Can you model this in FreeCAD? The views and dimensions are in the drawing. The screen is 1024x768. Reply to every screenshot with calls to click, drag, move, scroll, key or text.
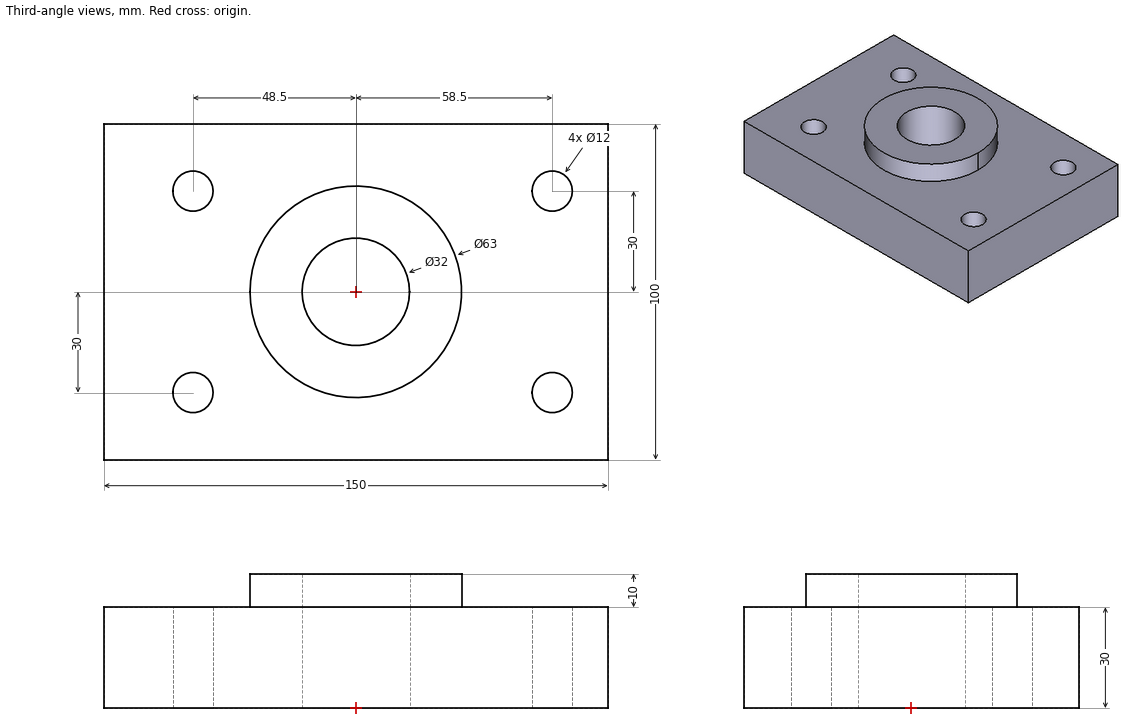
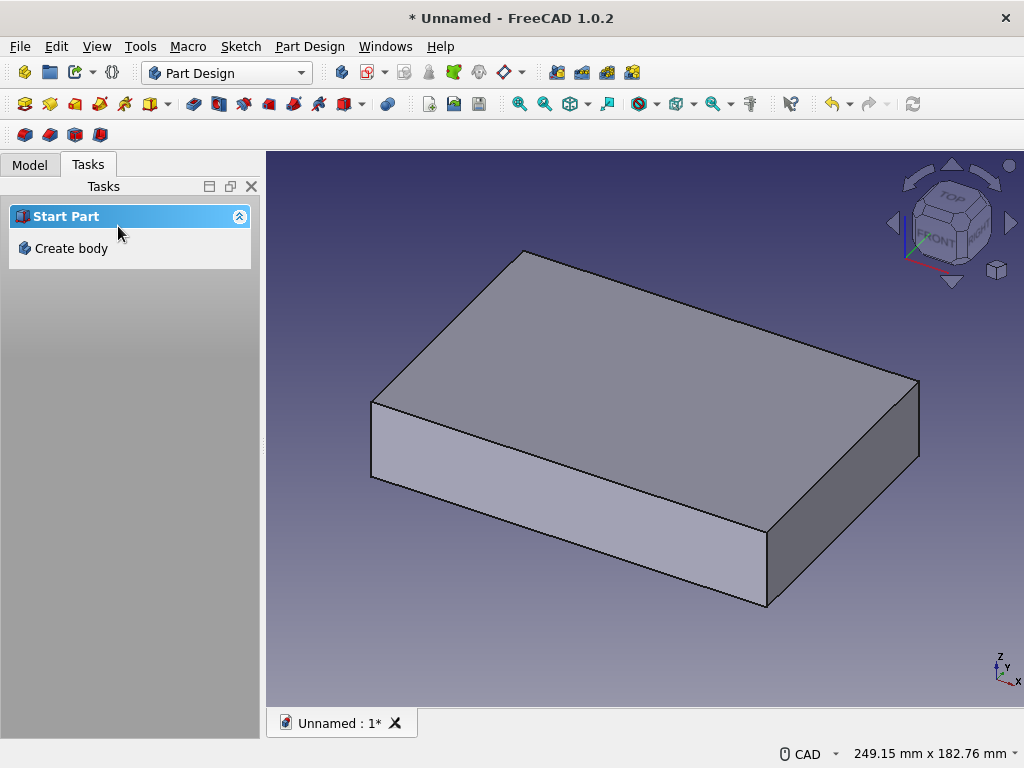
click(701, 409)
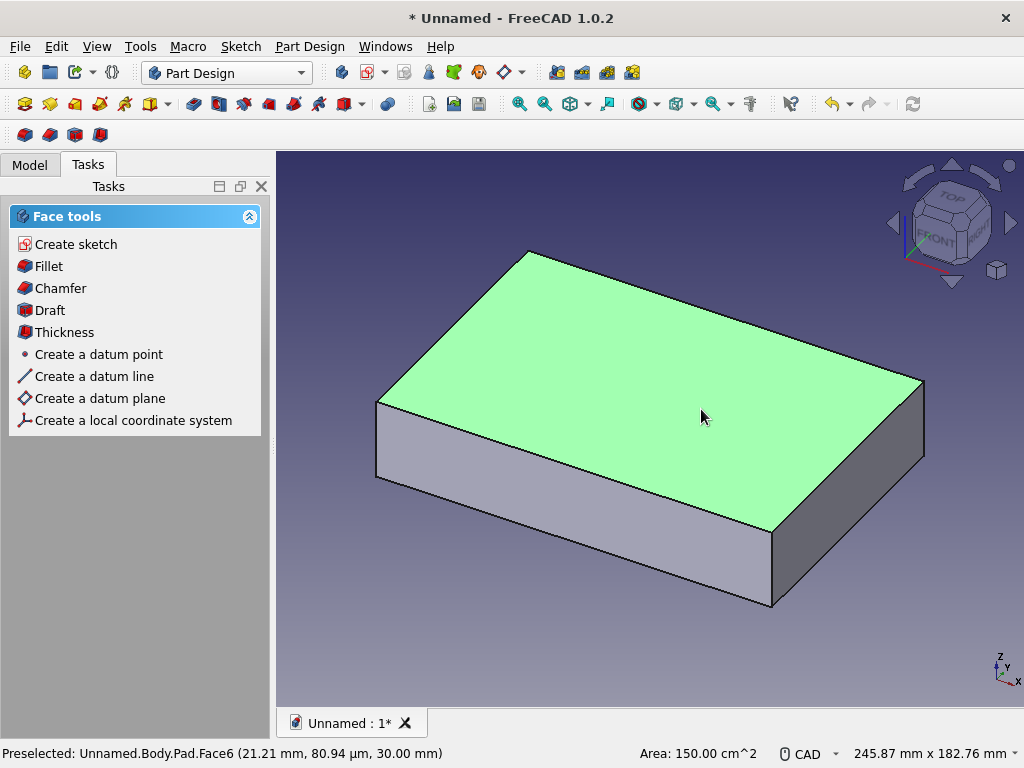
click(366, 72)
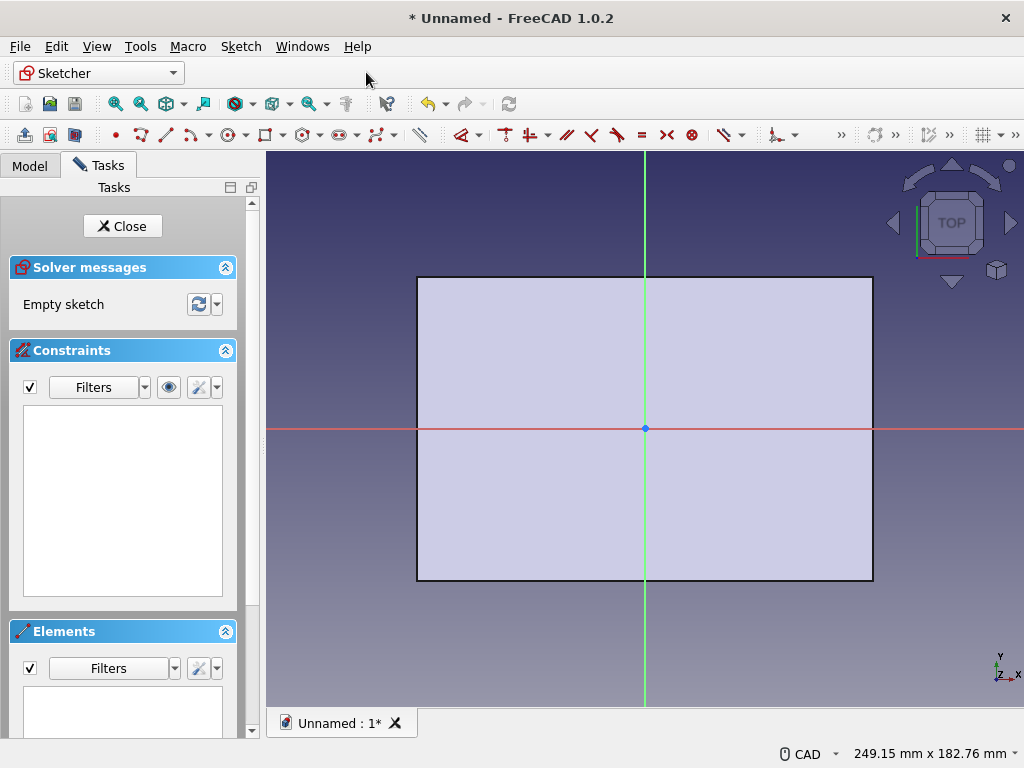
scroll(728, 429, up, 3)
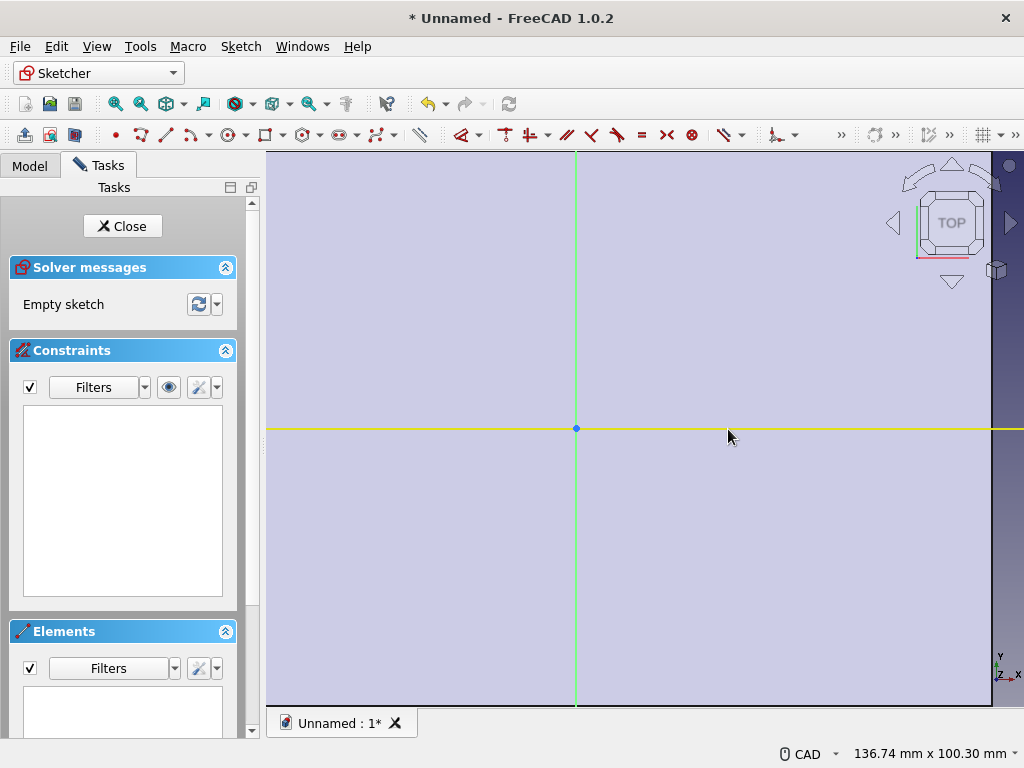
click(228, 136)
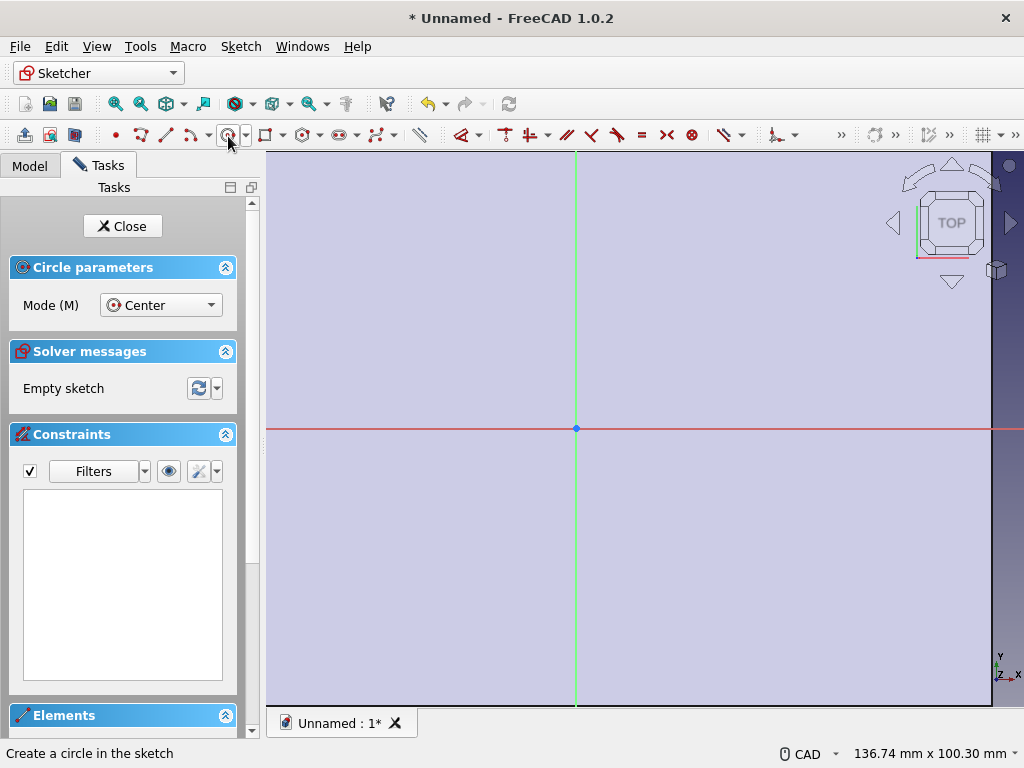
click(576, 429)
move(700, 305)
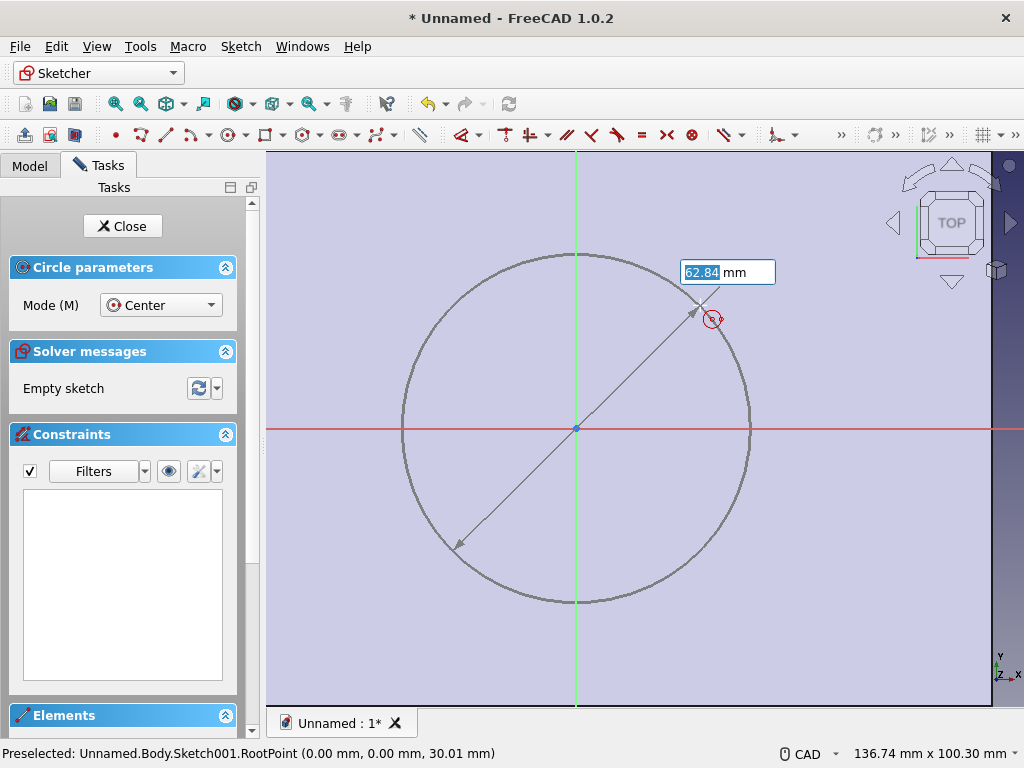
text(63)
key(Return)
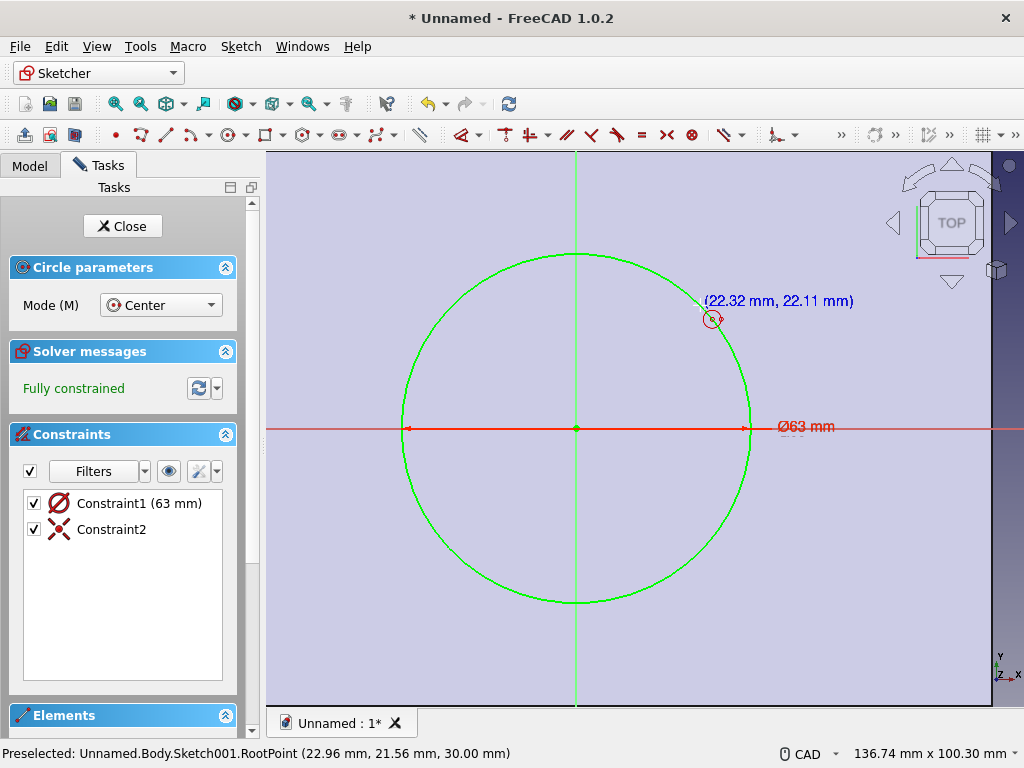
click(576, 429)
move(639, 366)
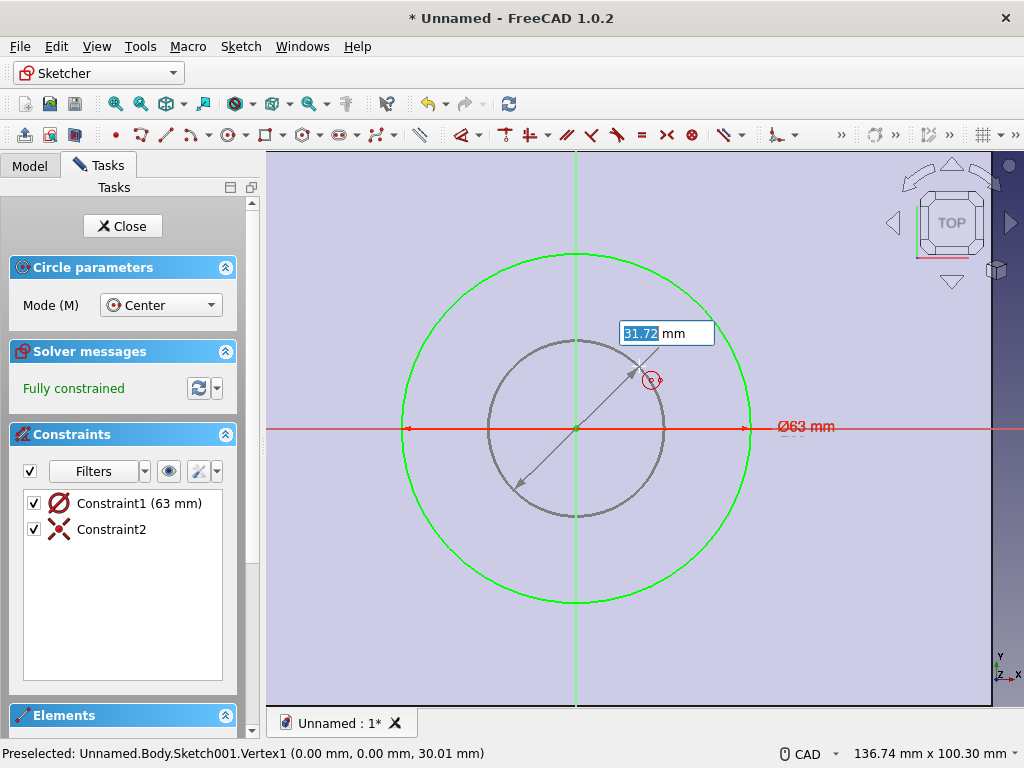
text(32)
key(Return)
key(Escape)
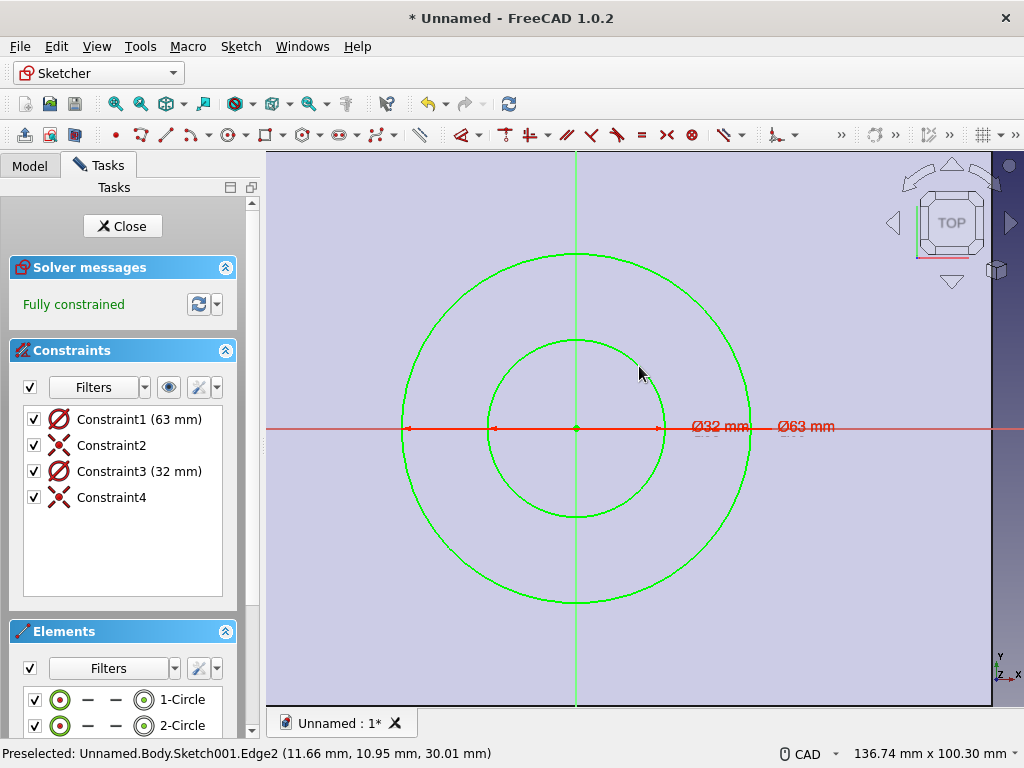
click(123, 226)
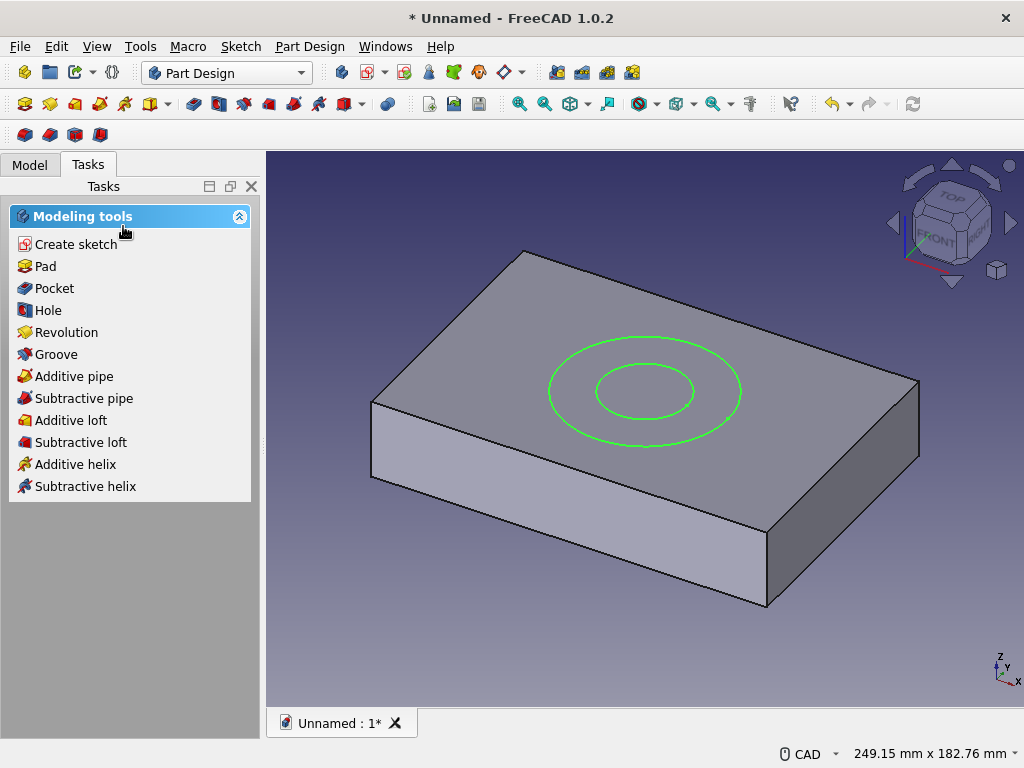
click(25, 104)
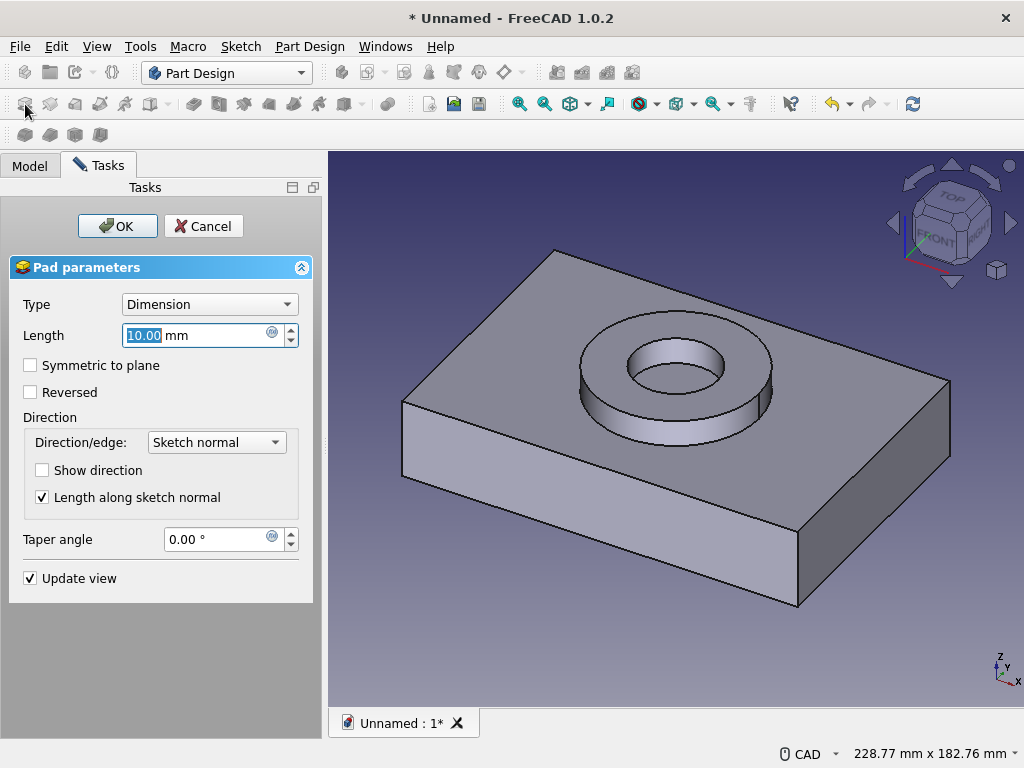
text(10)
key(Tab)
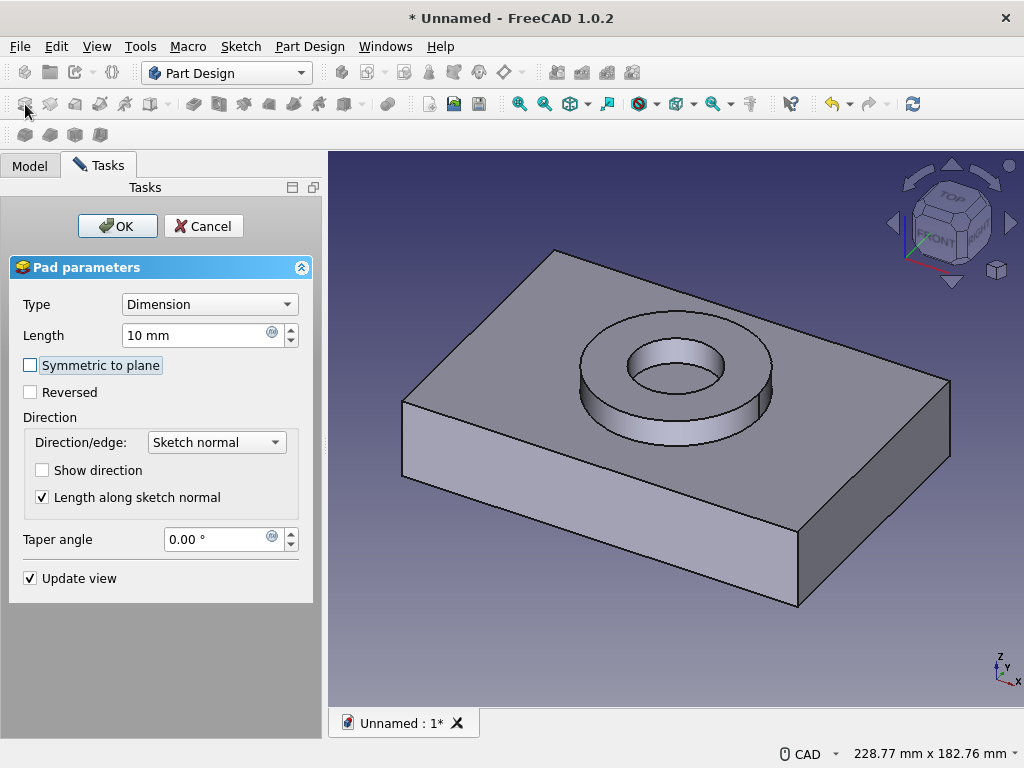
click(118, 226)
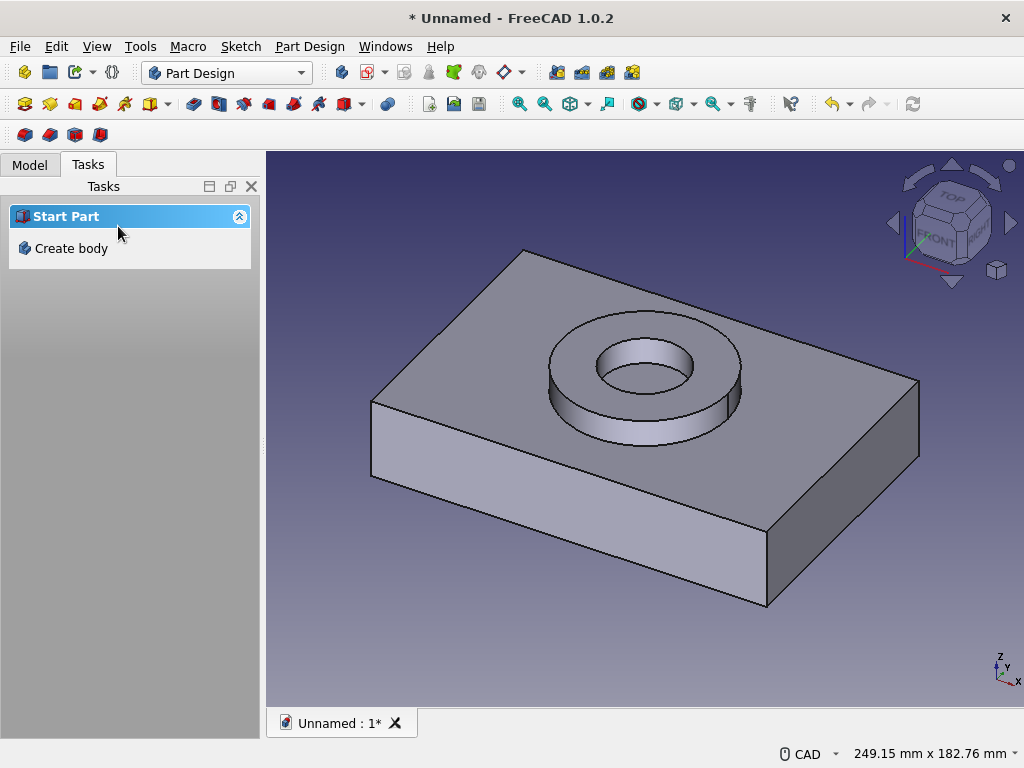
click(801, 384)